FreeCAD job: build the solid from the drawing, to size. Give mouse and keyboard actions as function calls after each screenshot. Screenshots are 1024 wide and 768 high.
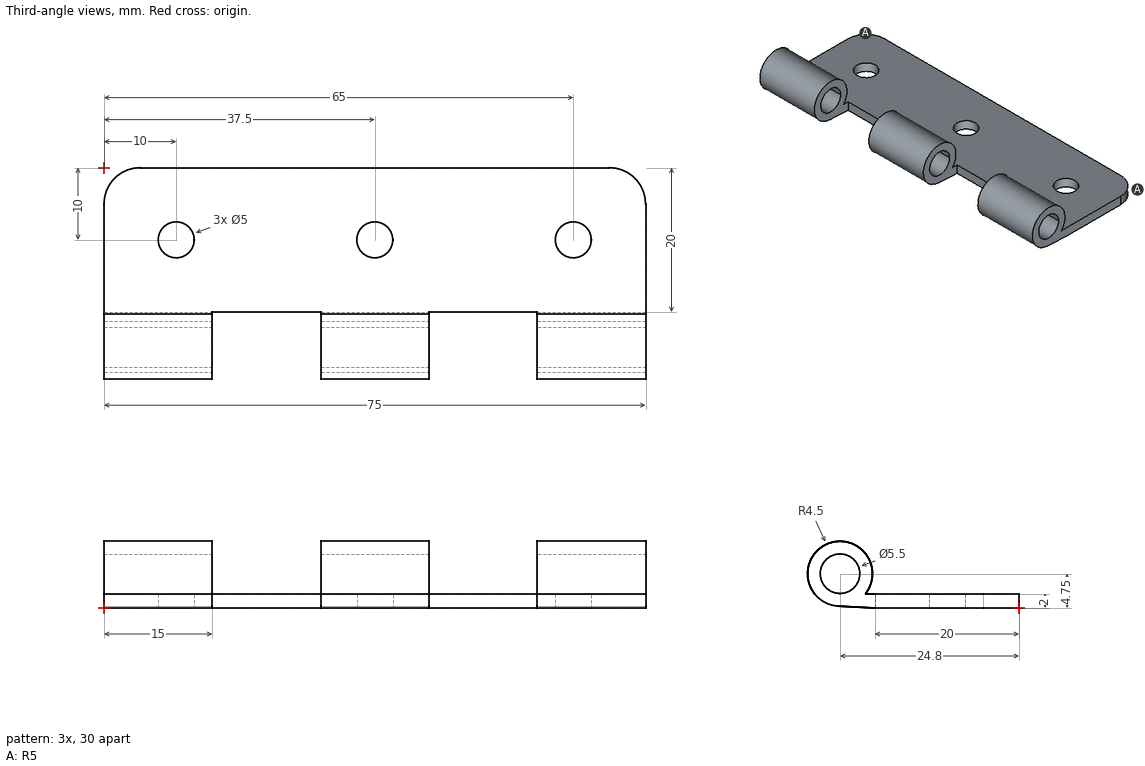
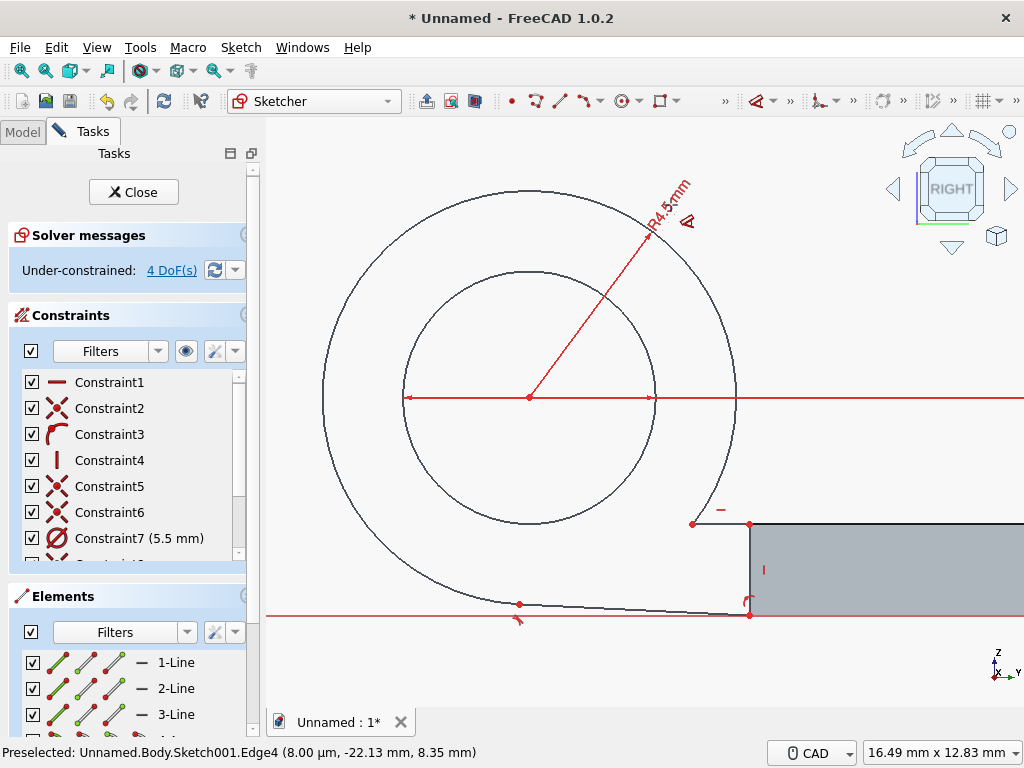
click(750, 552)
click(784, 570)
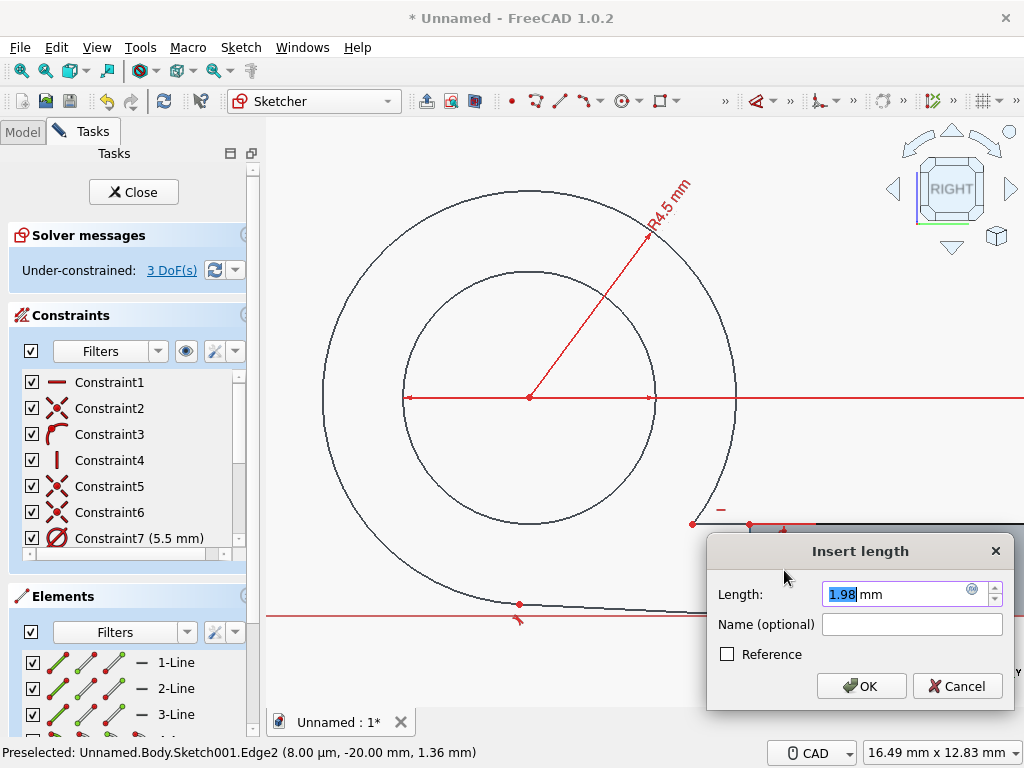
text(2)
key(Return)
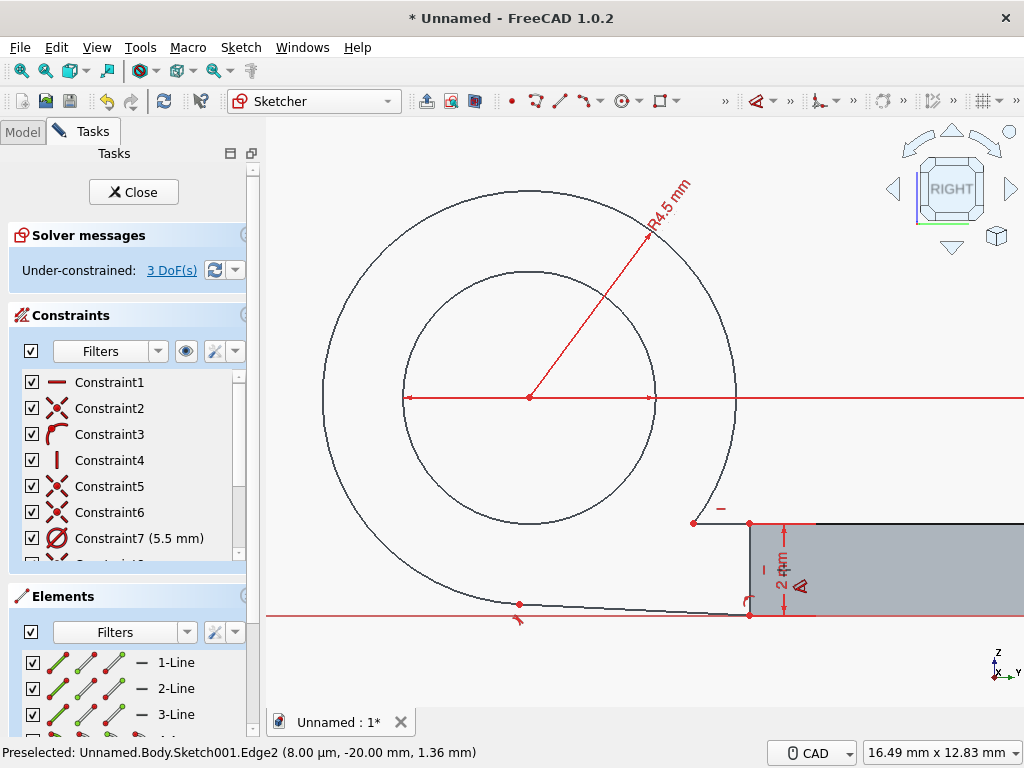
click(750, 524)
click(804, 650)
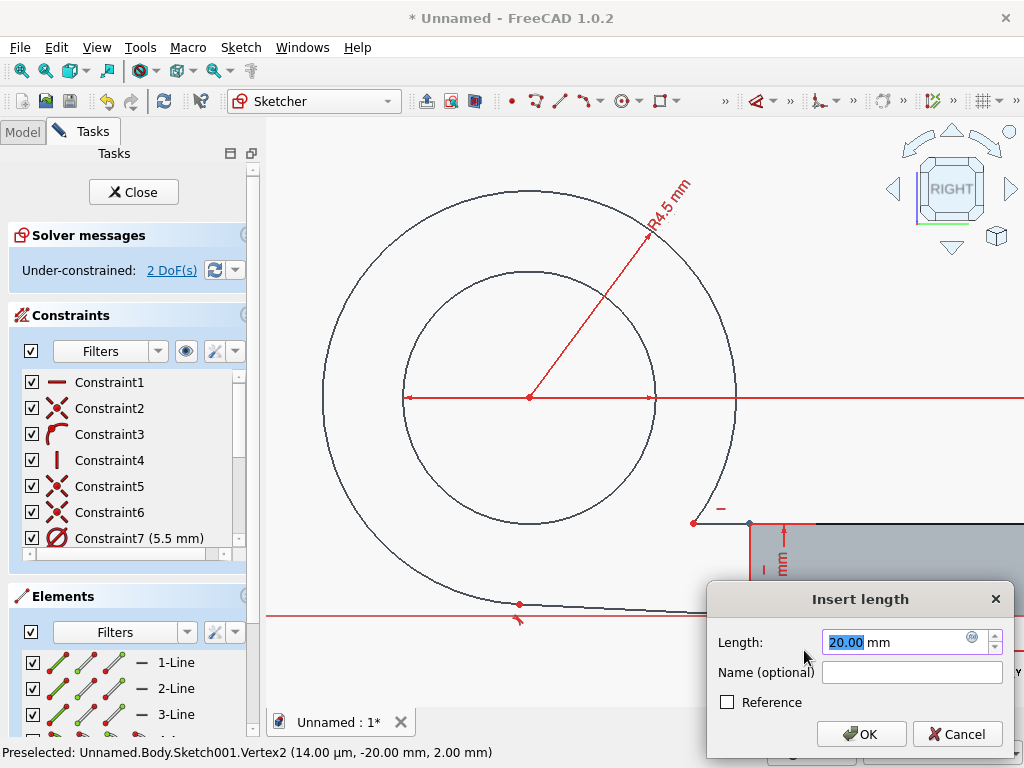
text(20)
key(Return)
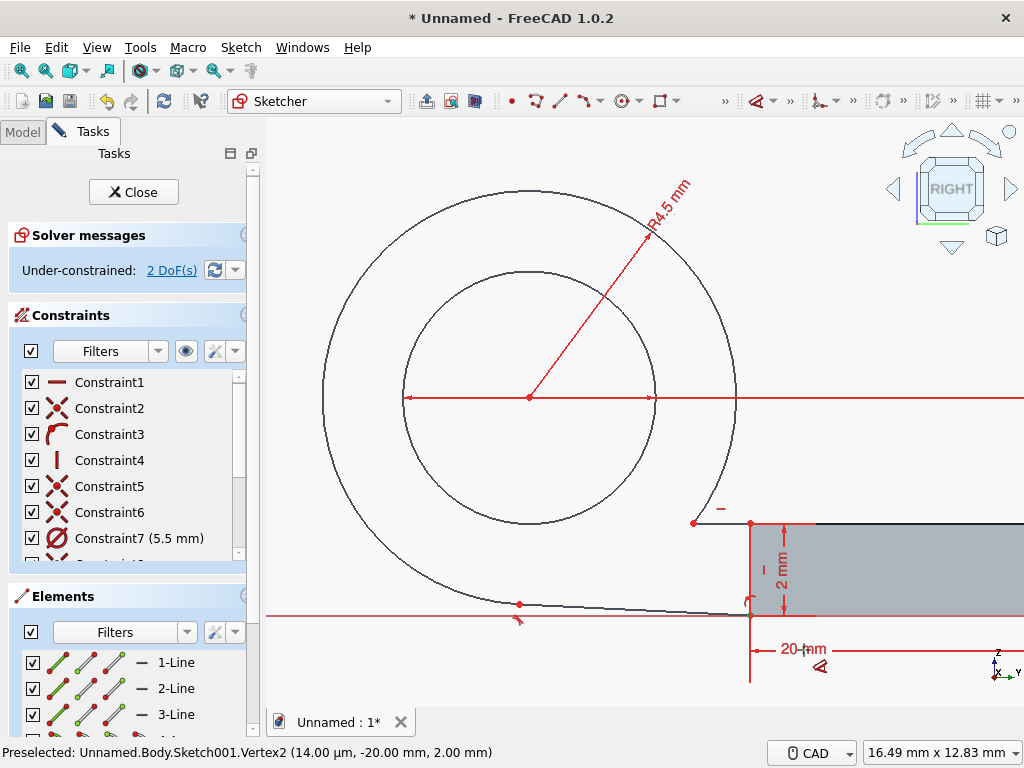
click(529, 398)
click(694, 650)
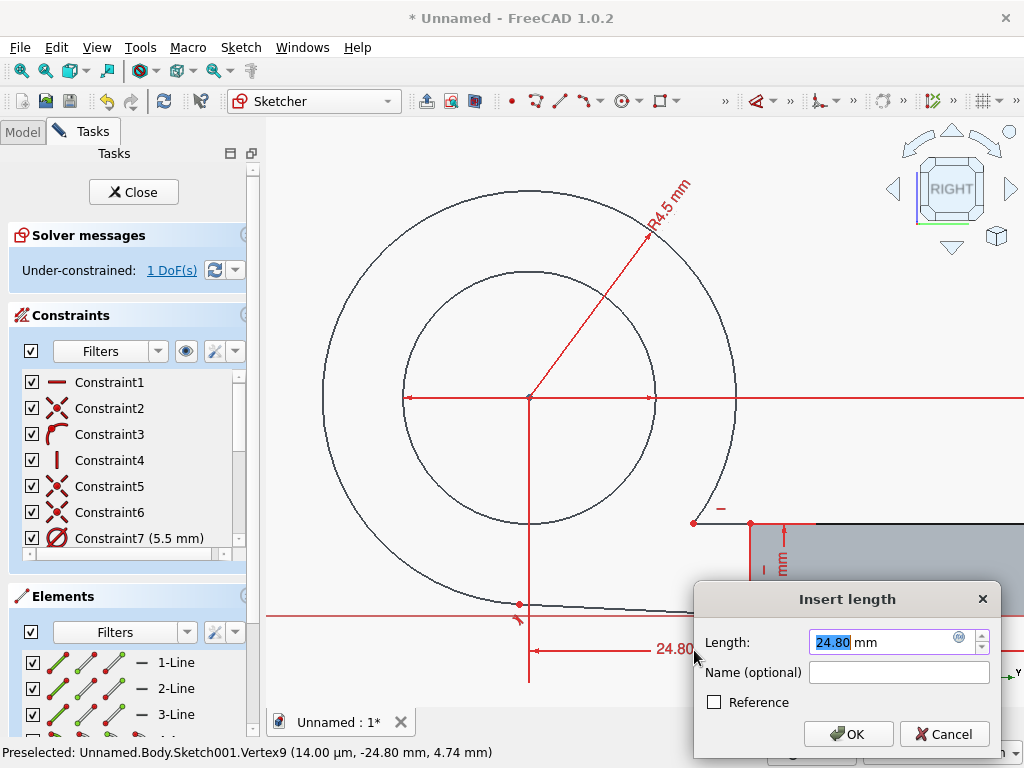
text(24.8)
key(Return)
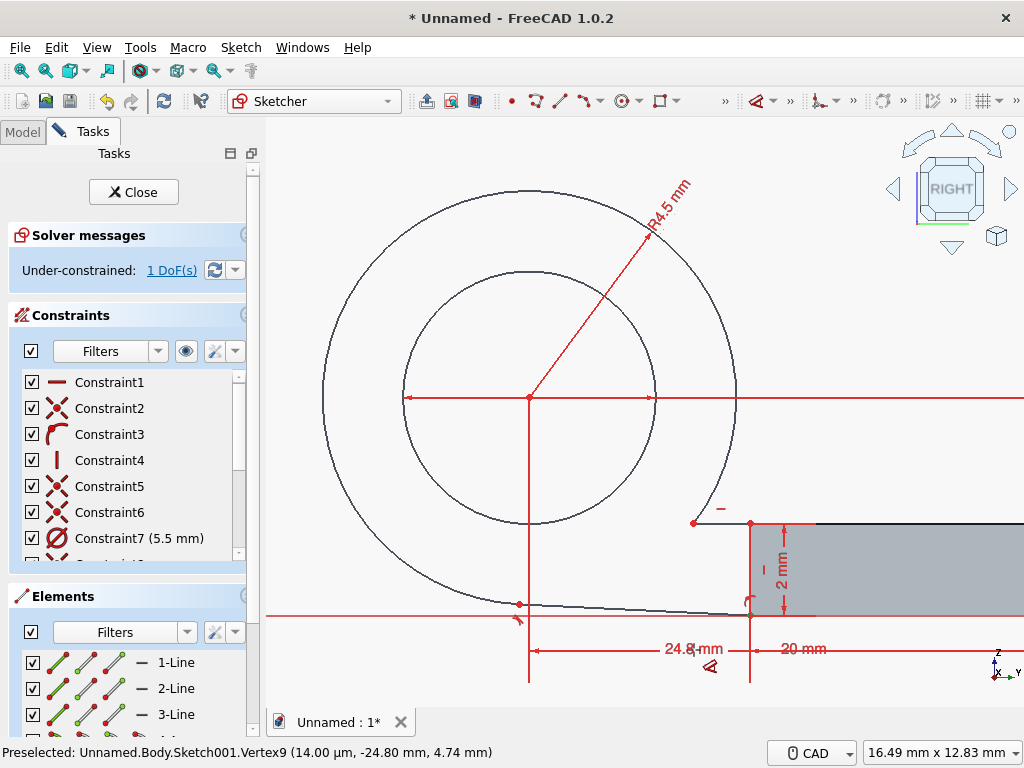
click(529, 398)
click(495, 457)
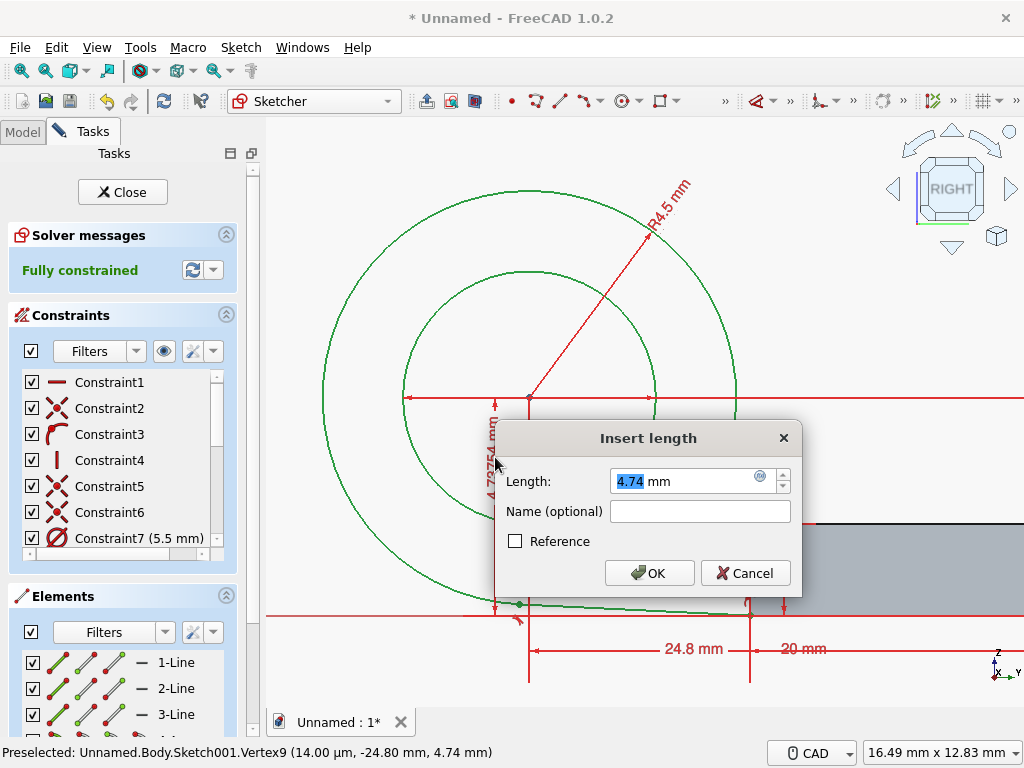
text(4.75)
key(Return)
key(Escape)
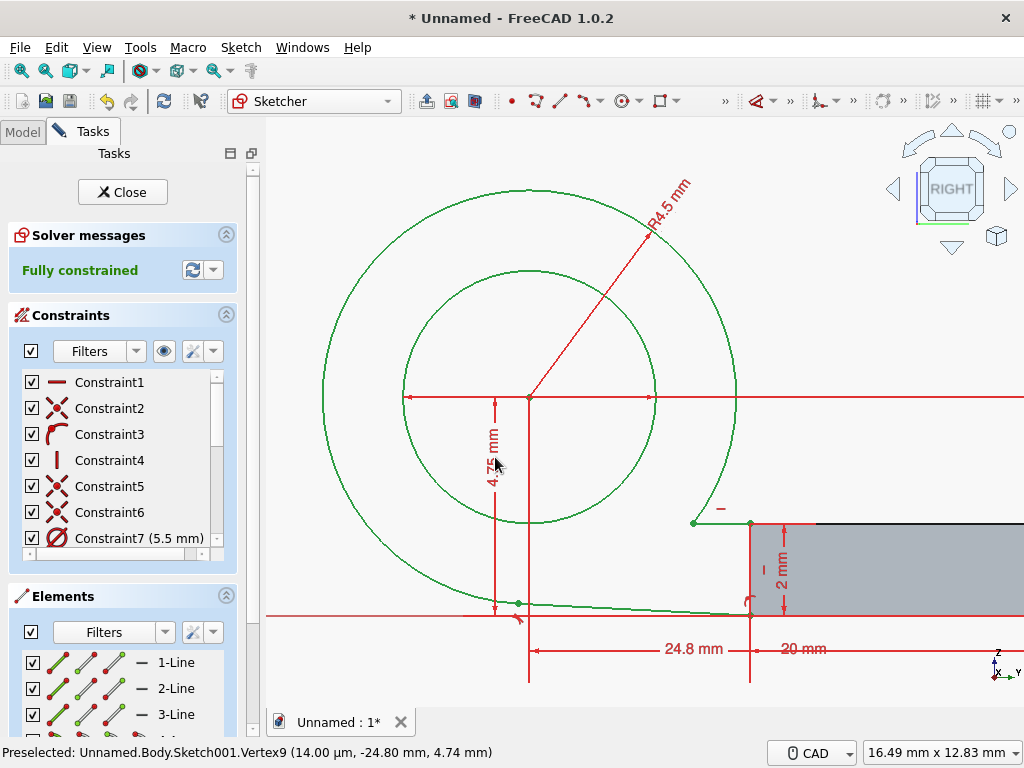
click(123, 192)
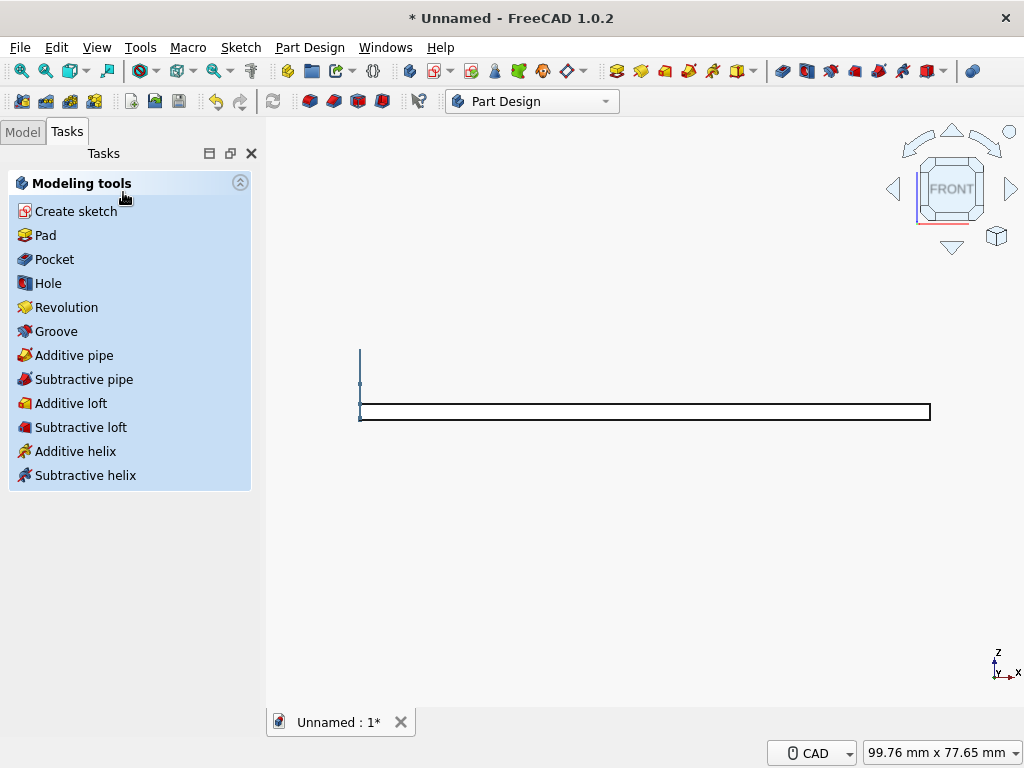
click(618, 72)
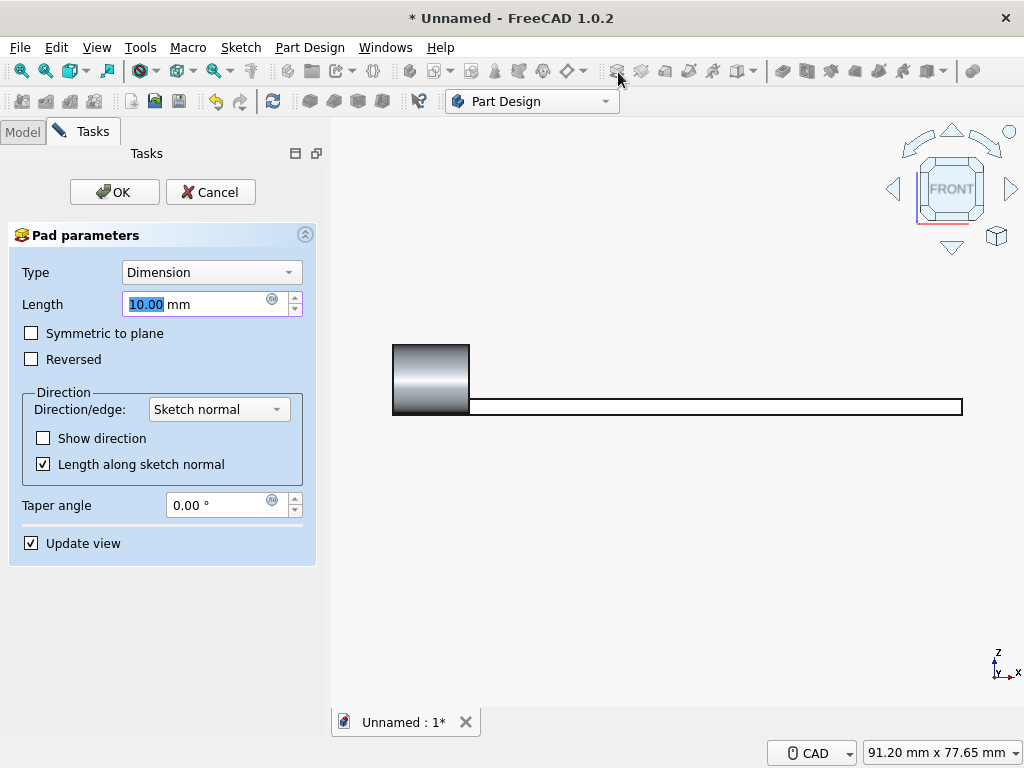
text(15)
key(Tab)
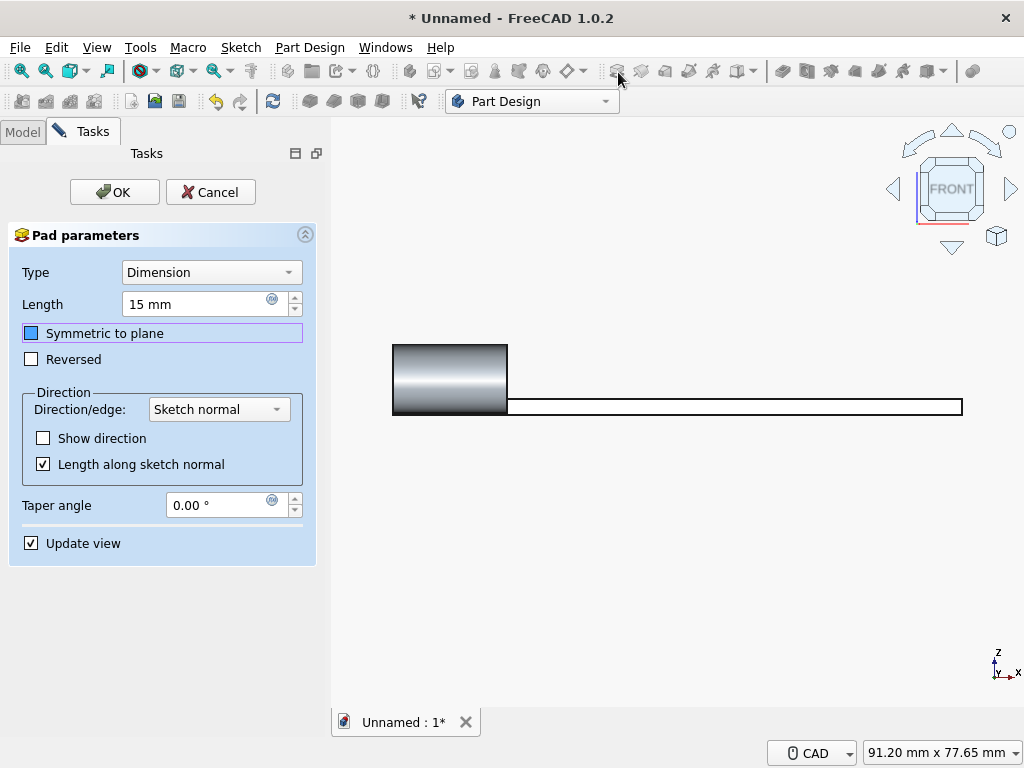
click(115, 192)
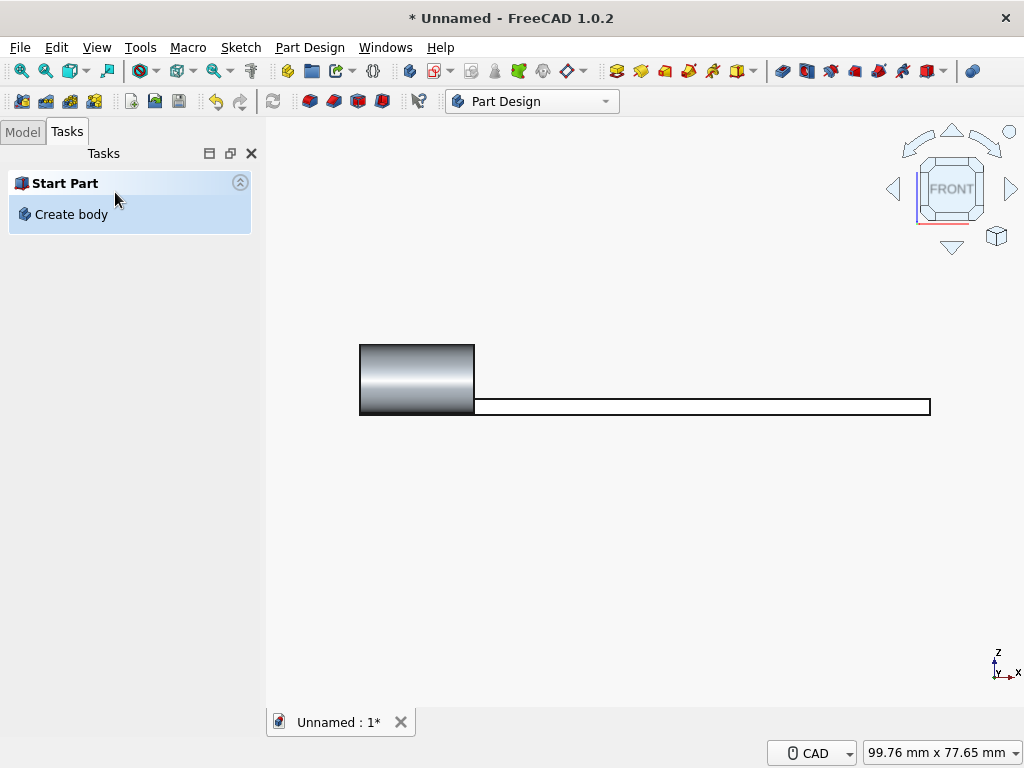
click(23, 131)